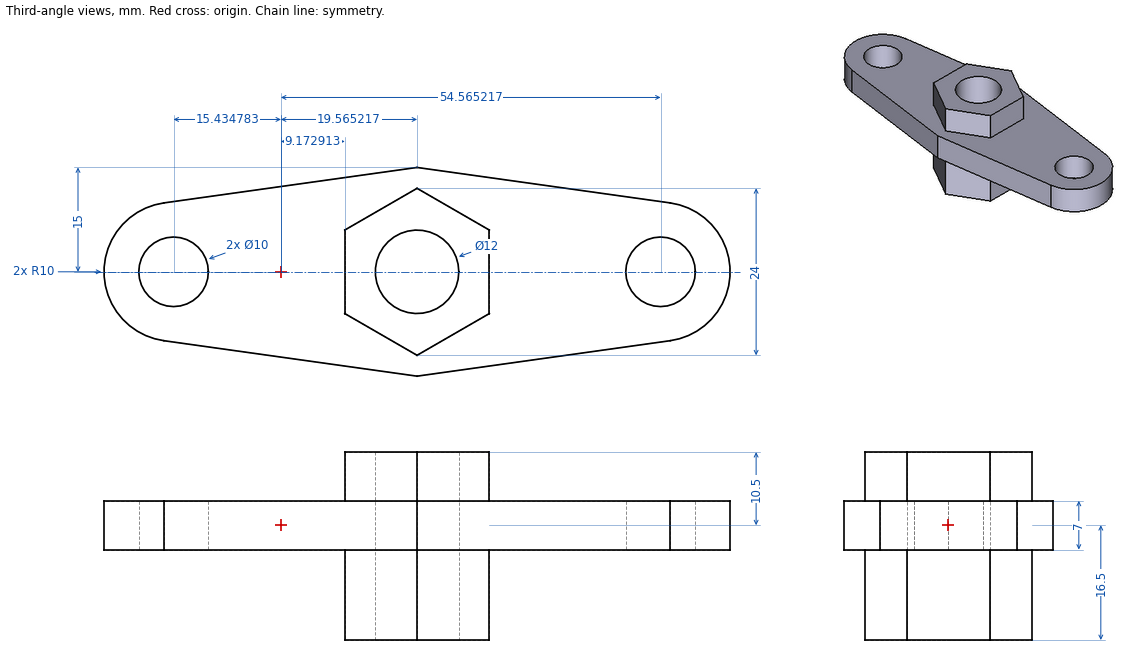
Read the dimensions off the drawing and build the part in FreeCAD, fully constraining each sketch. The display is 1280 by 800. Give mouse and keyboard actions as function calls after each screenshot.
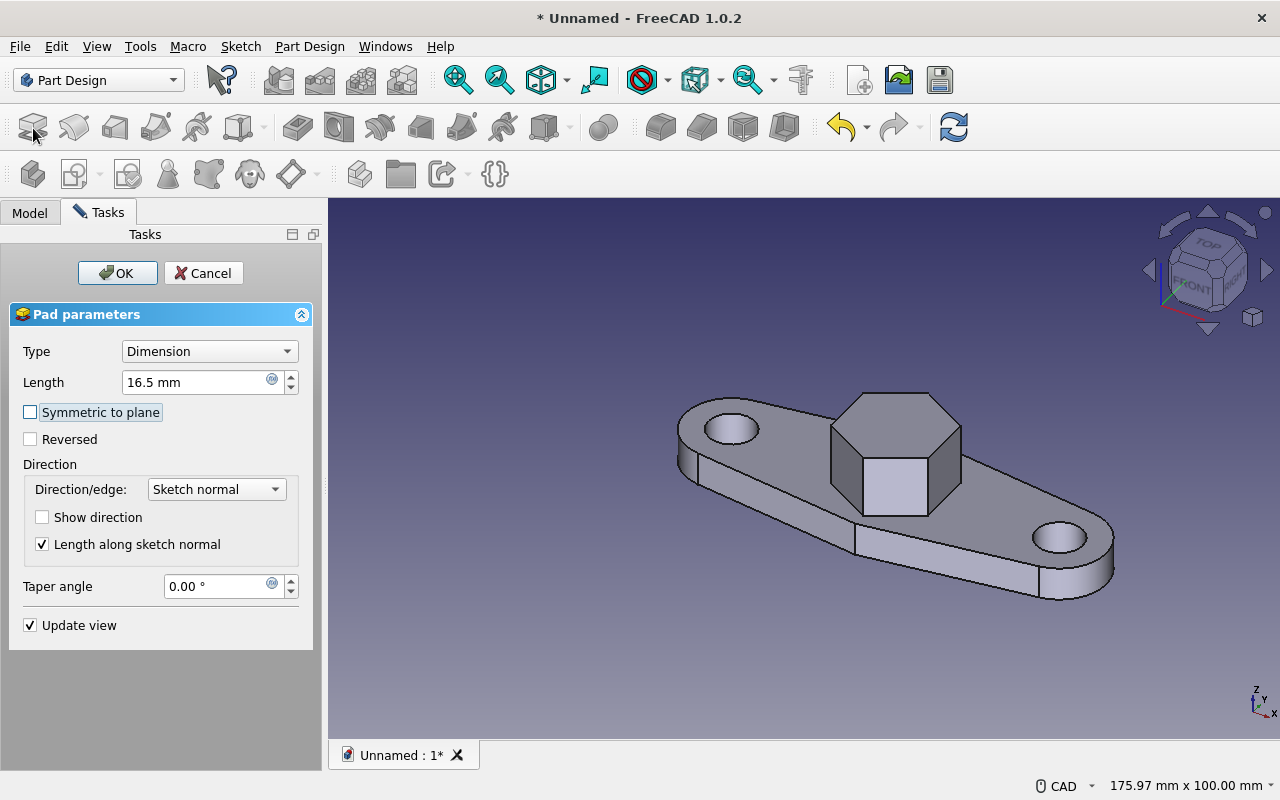
click(31, 439)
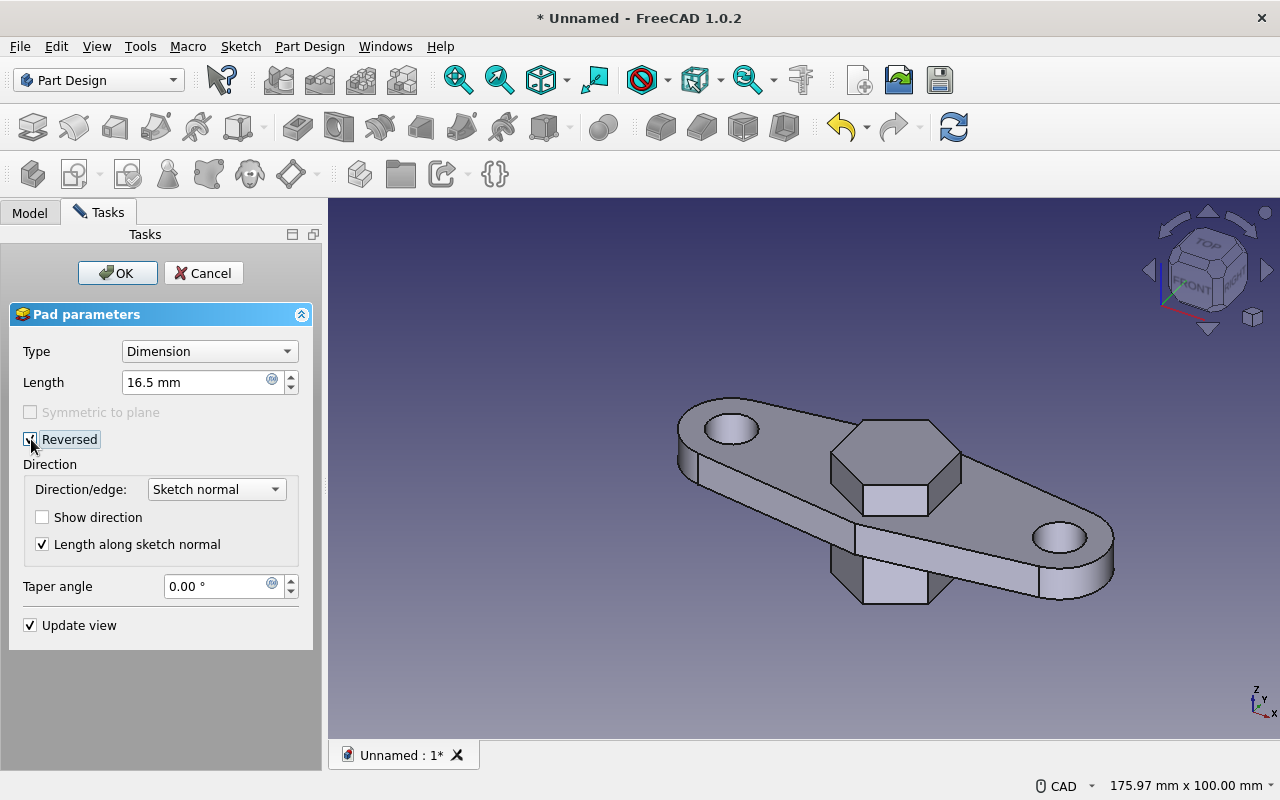
click(118, 273)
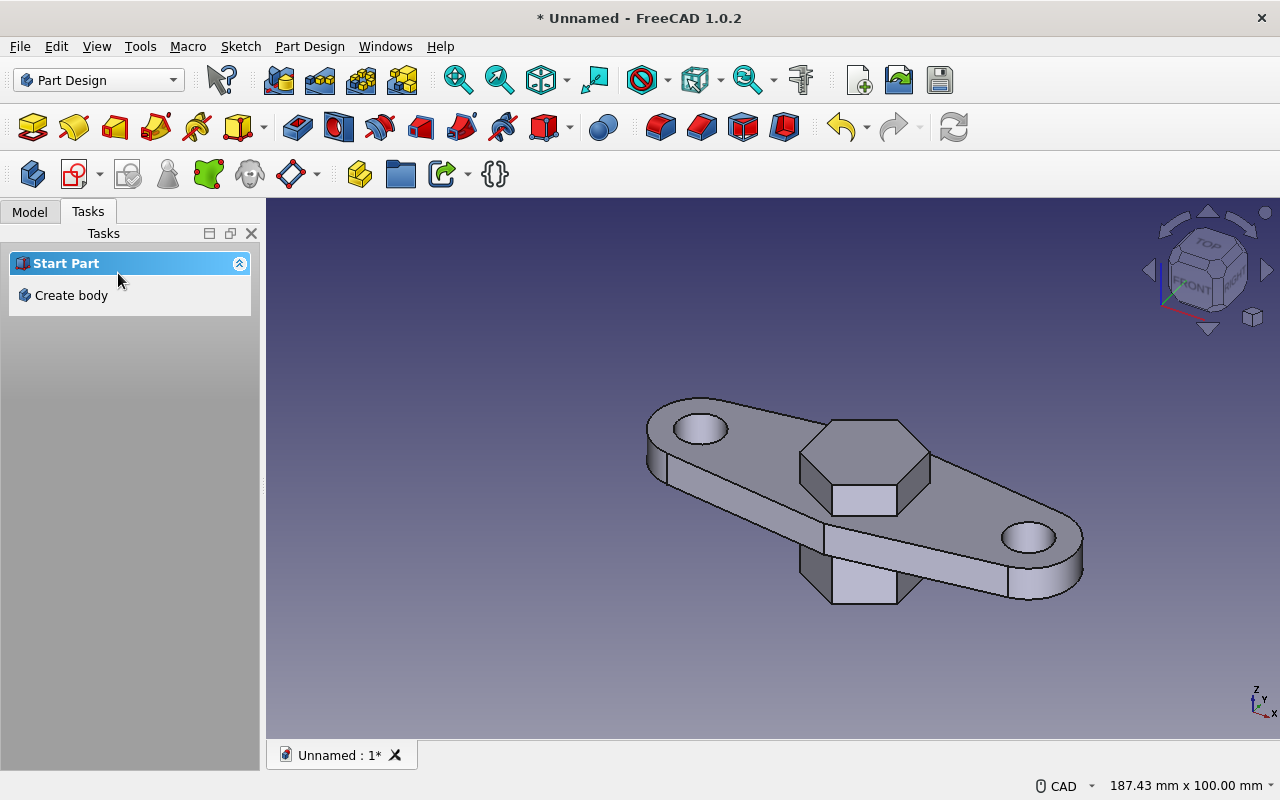
click(865, 451)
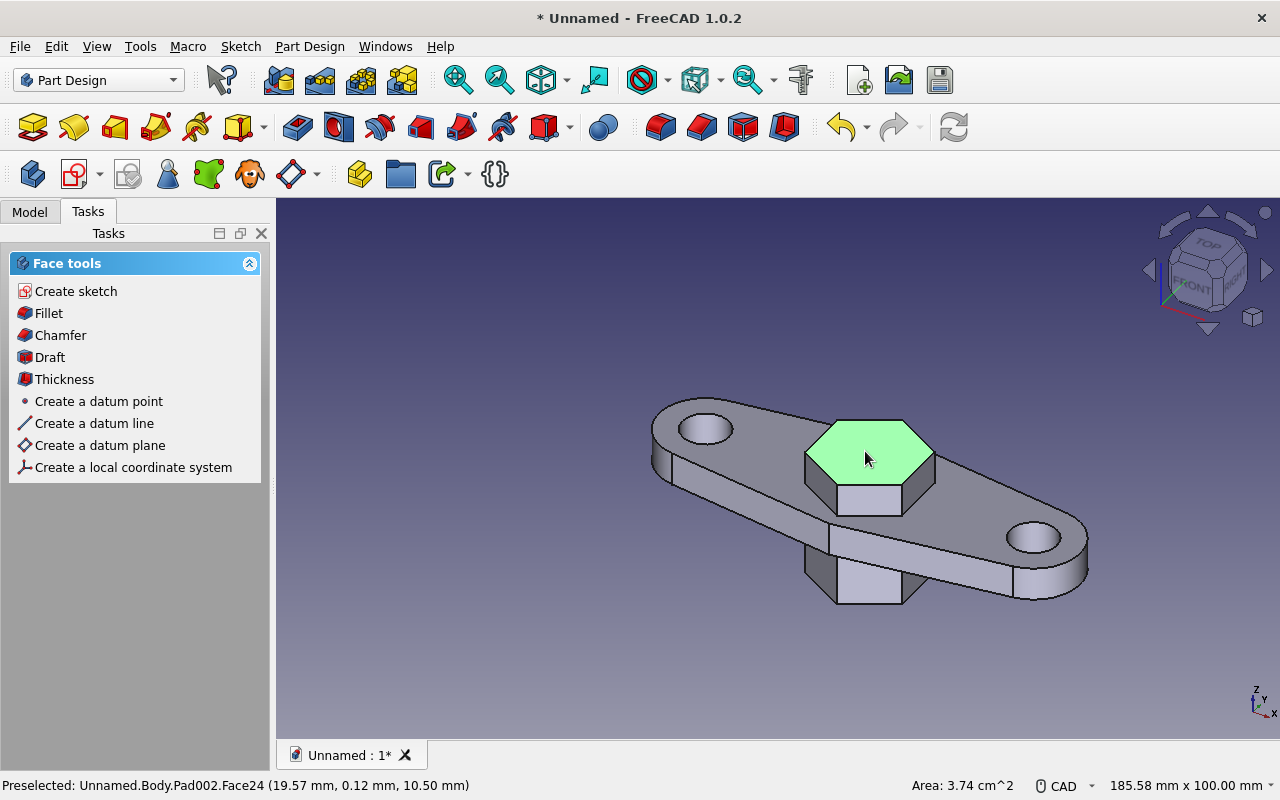
click(74, 174)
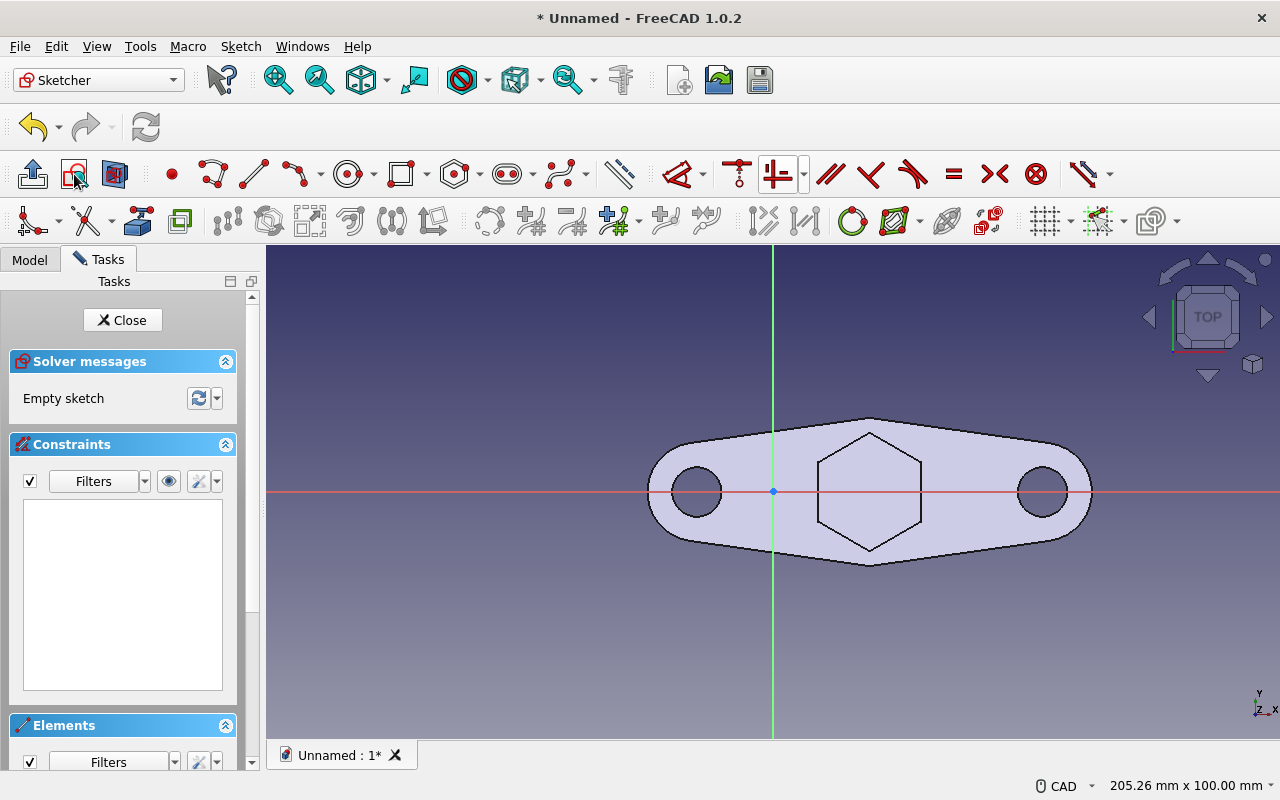
scroll(869, 492, up, 8)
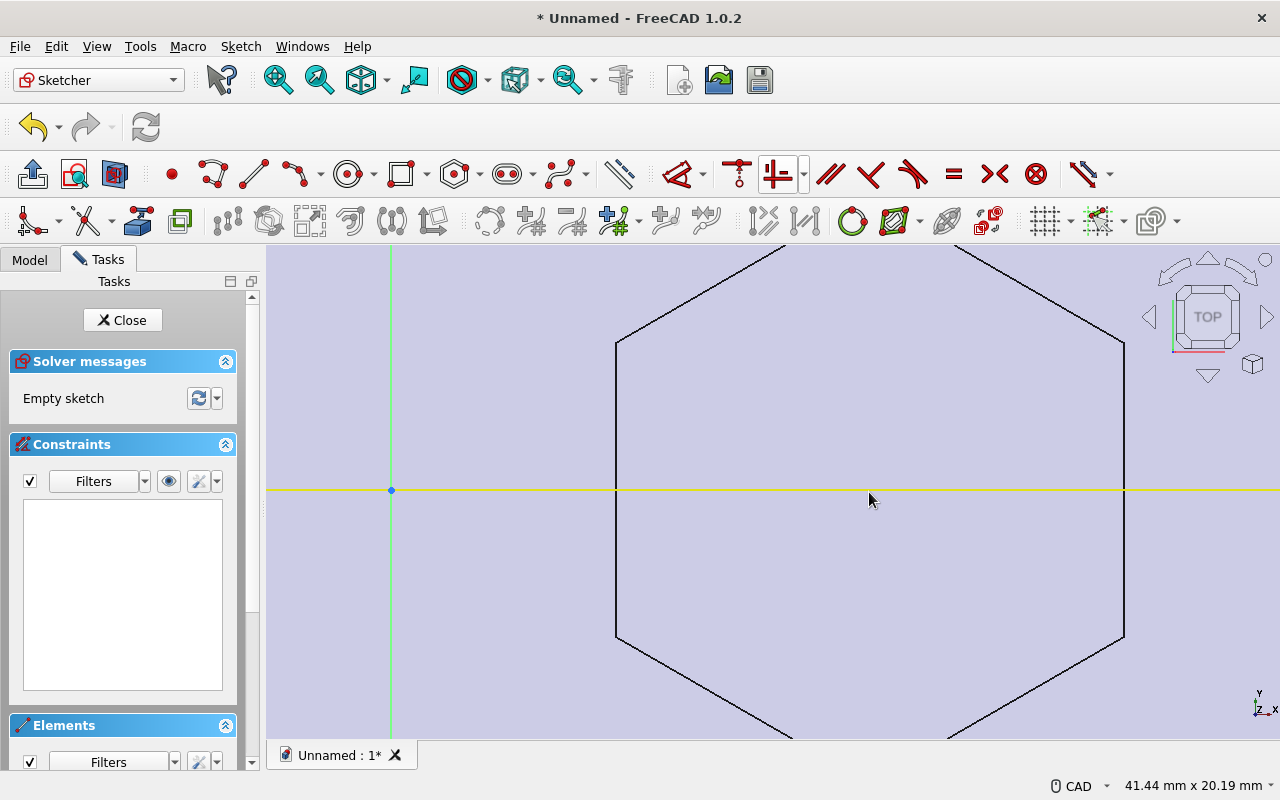
click(348, 174)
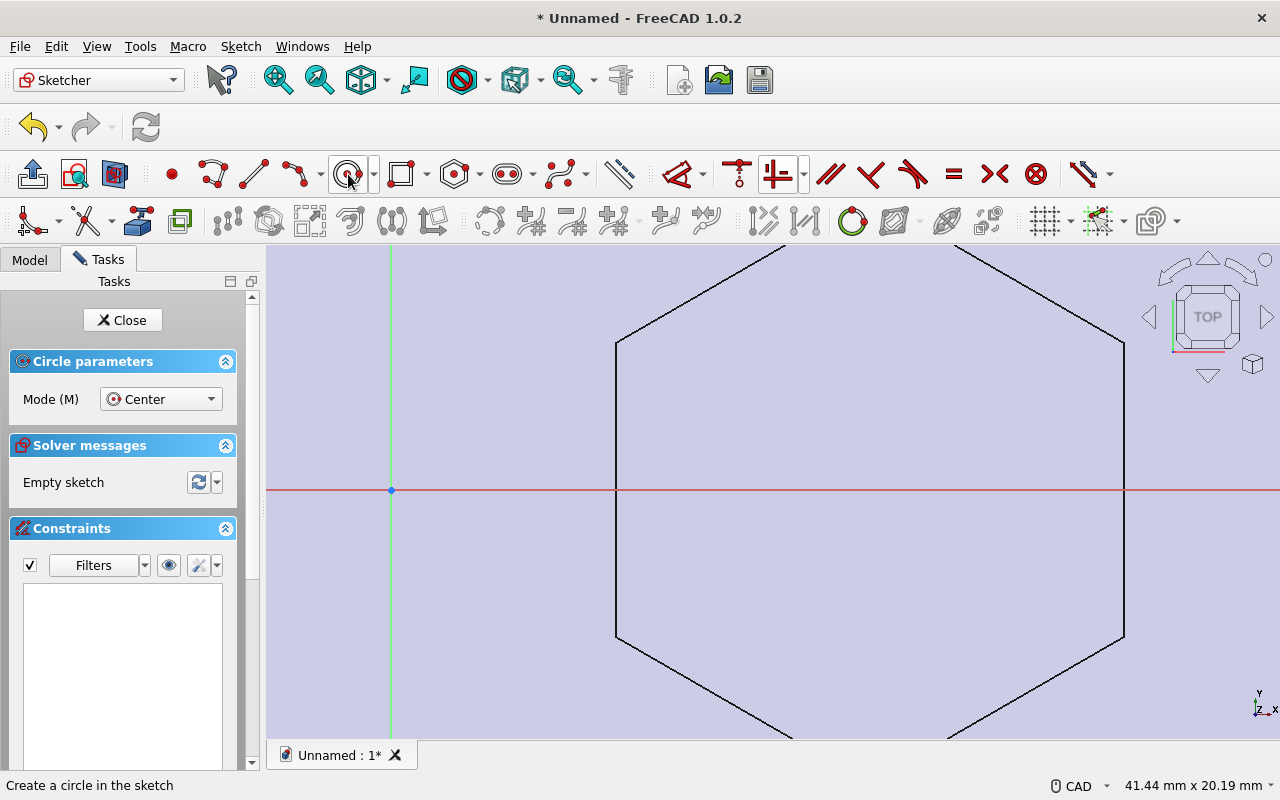
click(870, 490)
move(974, 386)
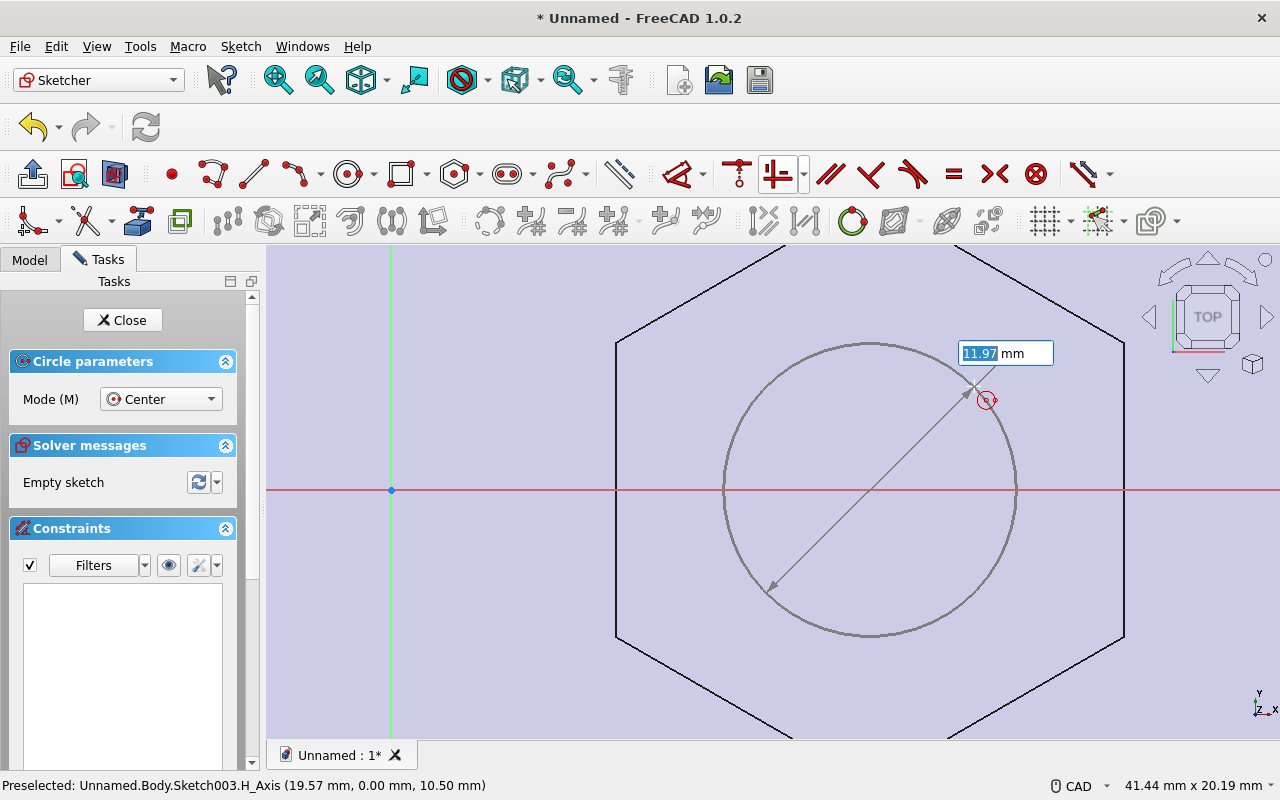
text(12)
key(Return)
key(Escape)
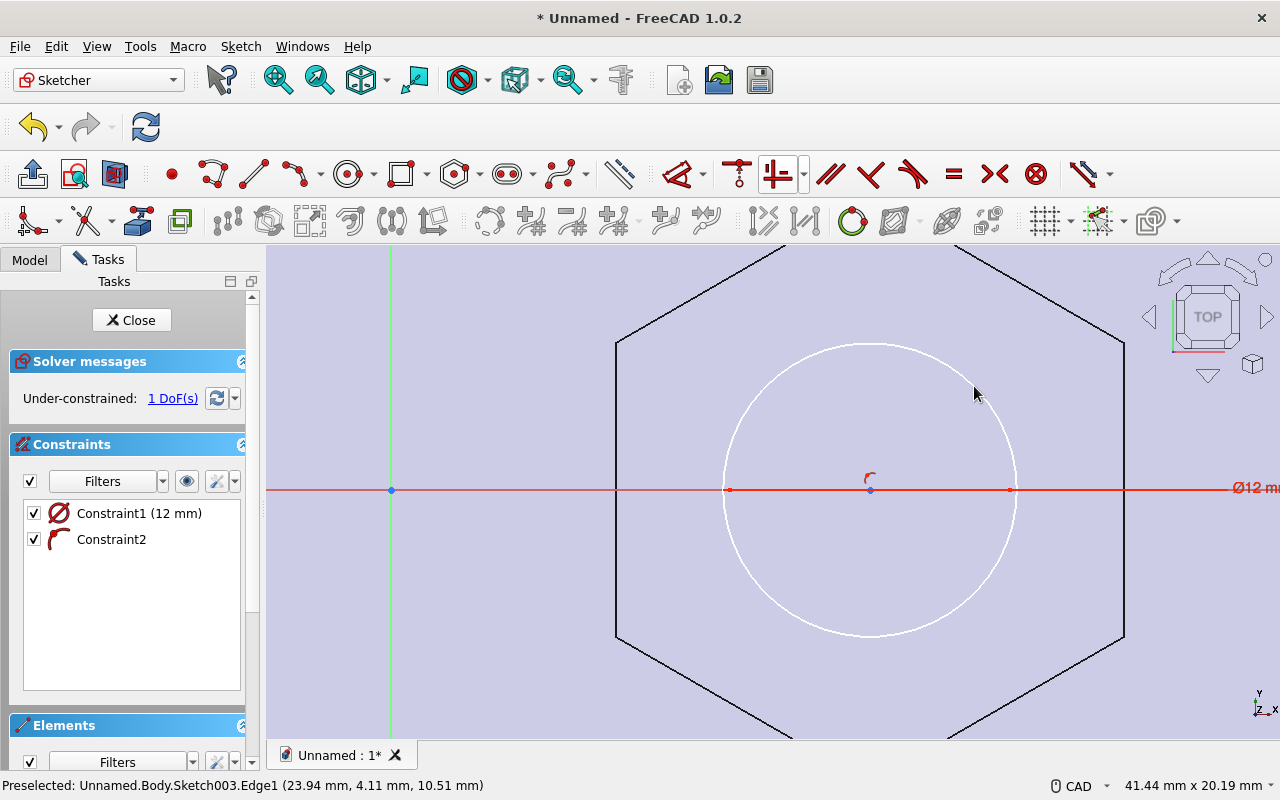
click(676, 174)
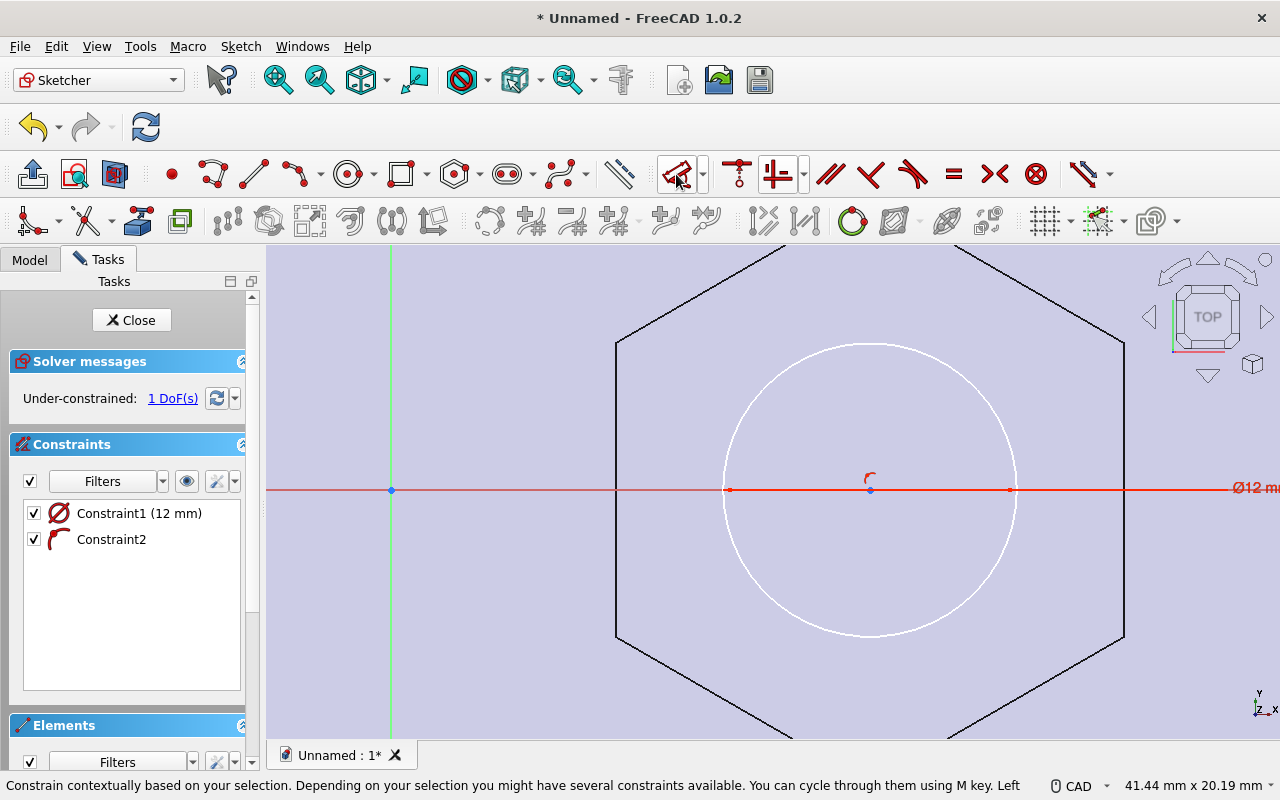
click(870, 490)
click(631, 524)